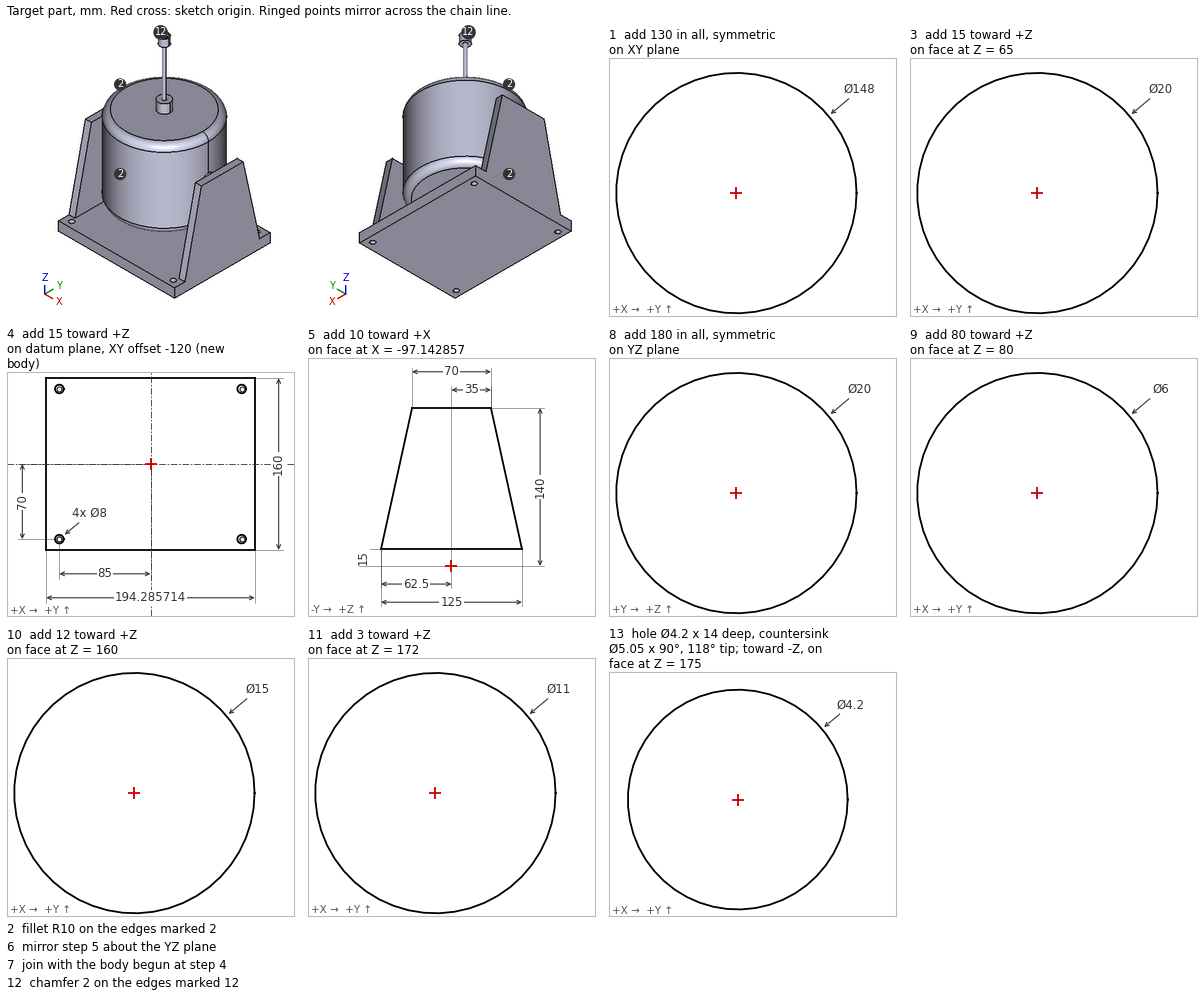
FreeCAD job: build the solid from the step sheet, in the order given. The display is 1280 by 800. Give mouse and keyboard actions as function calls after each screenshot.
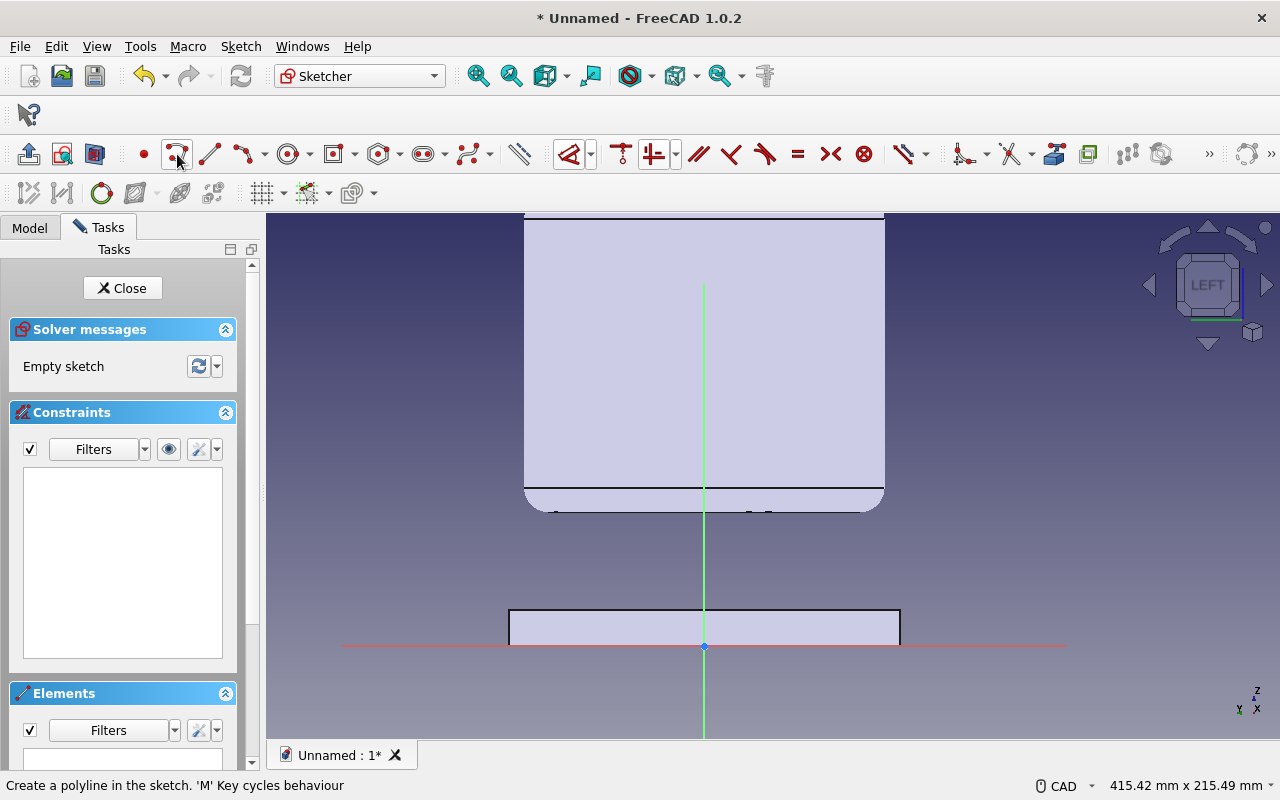
click(552, 610)
click(857, 610)
click(790, 305)
click(619, 305)
click(552, 611)
key(Escape)
key(Escape)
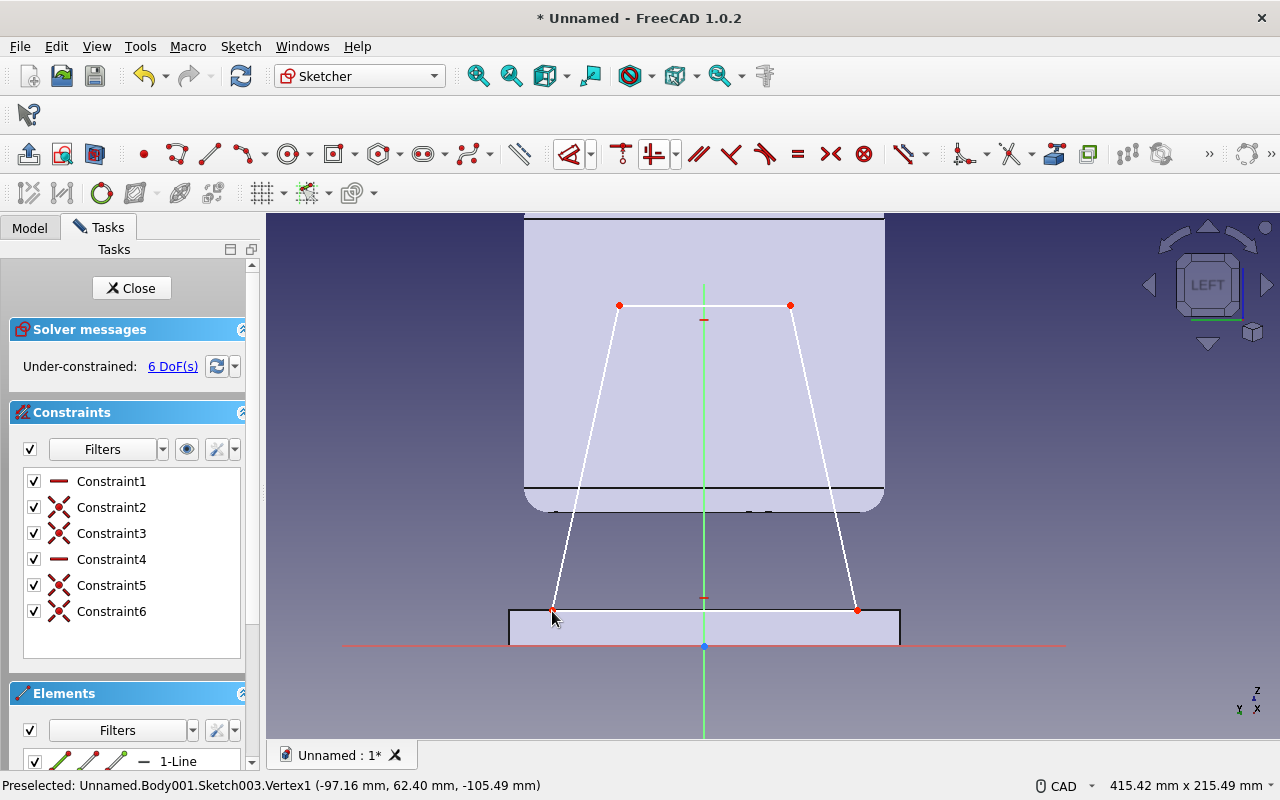
click(739, 306)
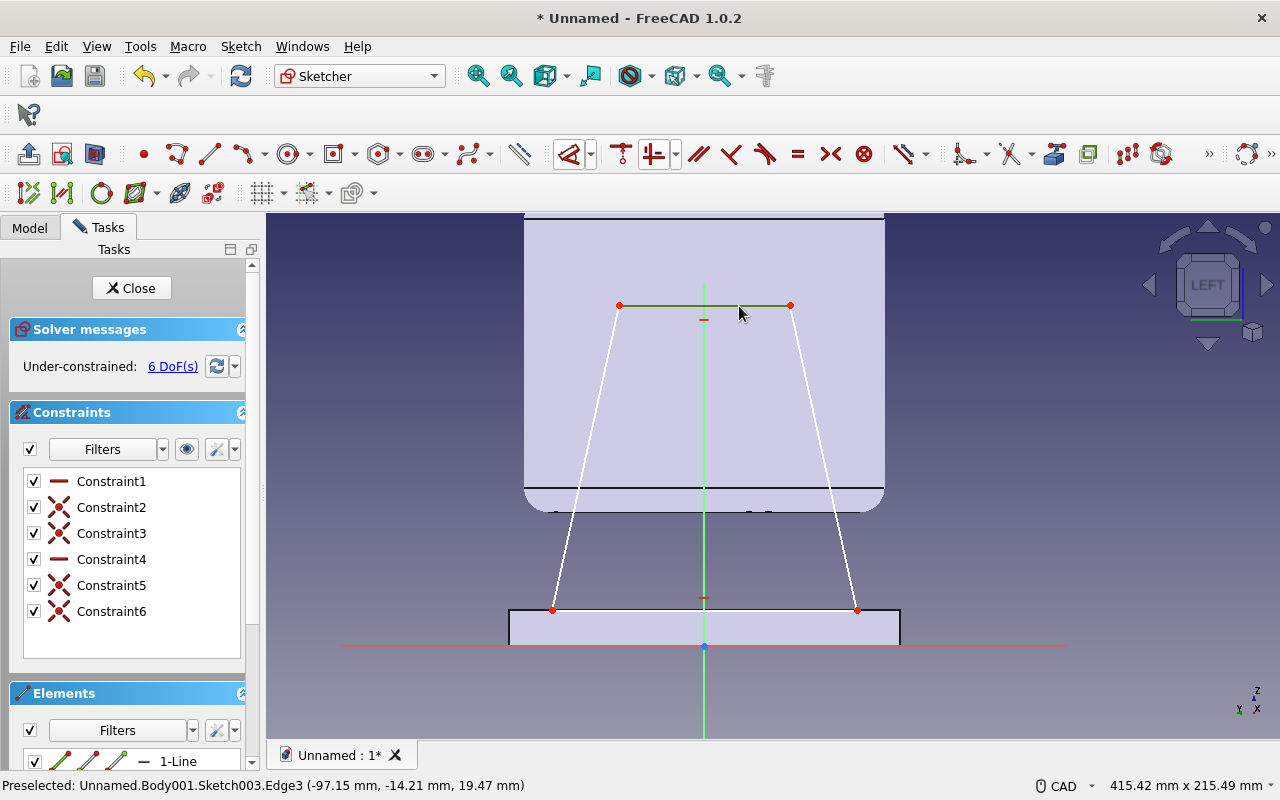
key(l)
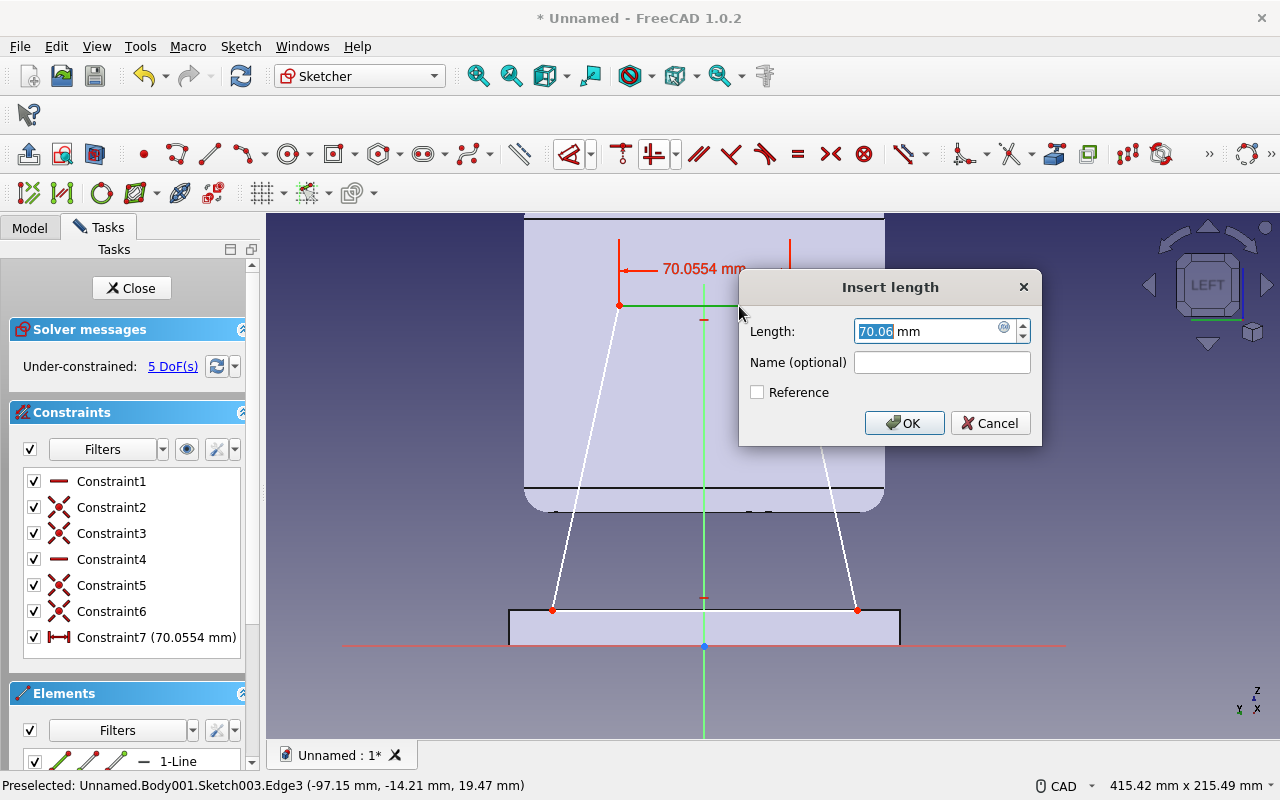
text(70)
key(Return)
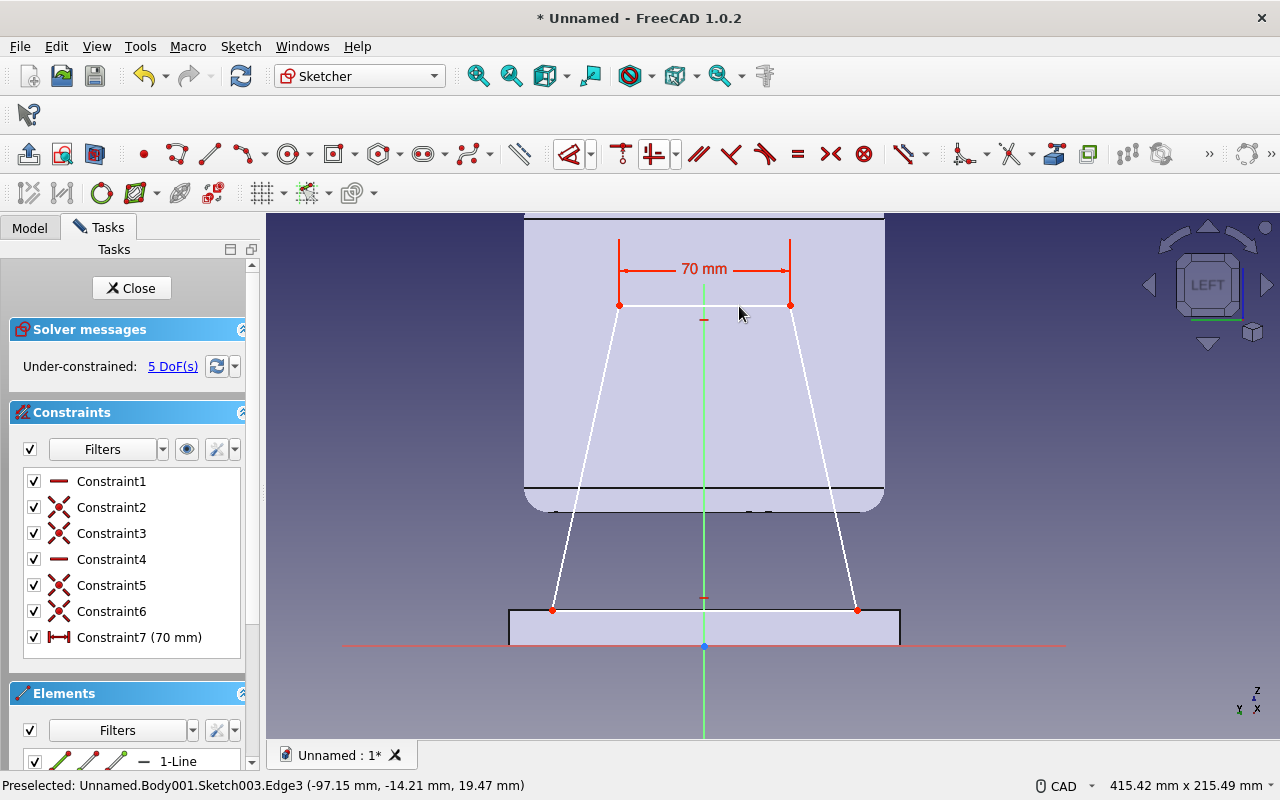
click(644, 611)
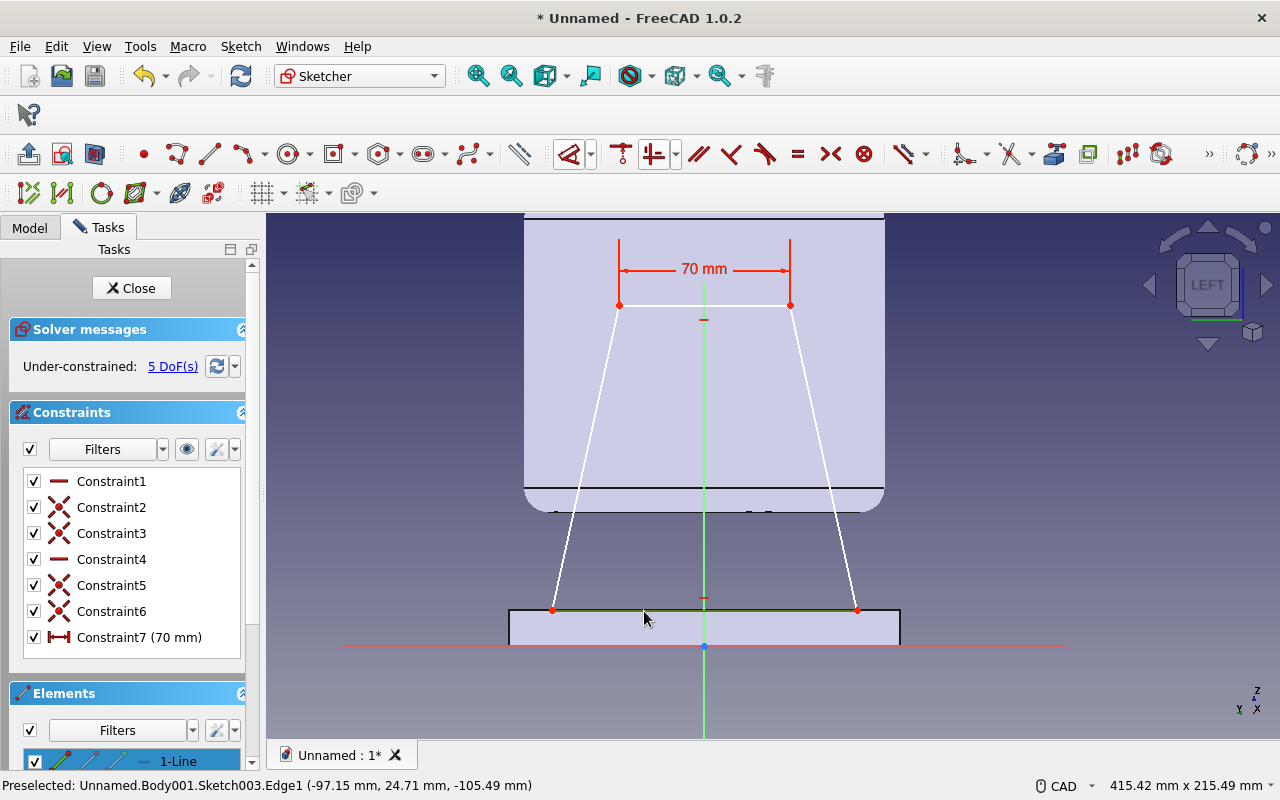
key(l)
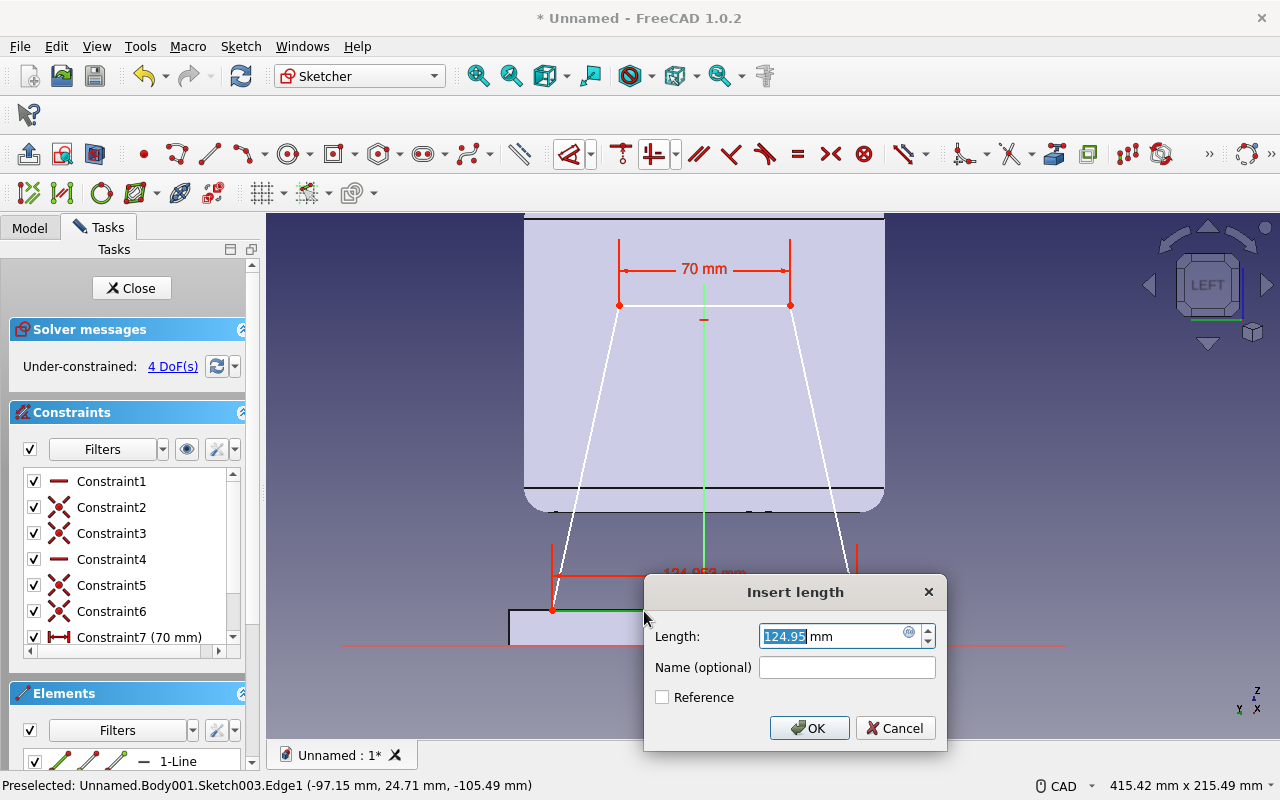
text(125)
key(Return)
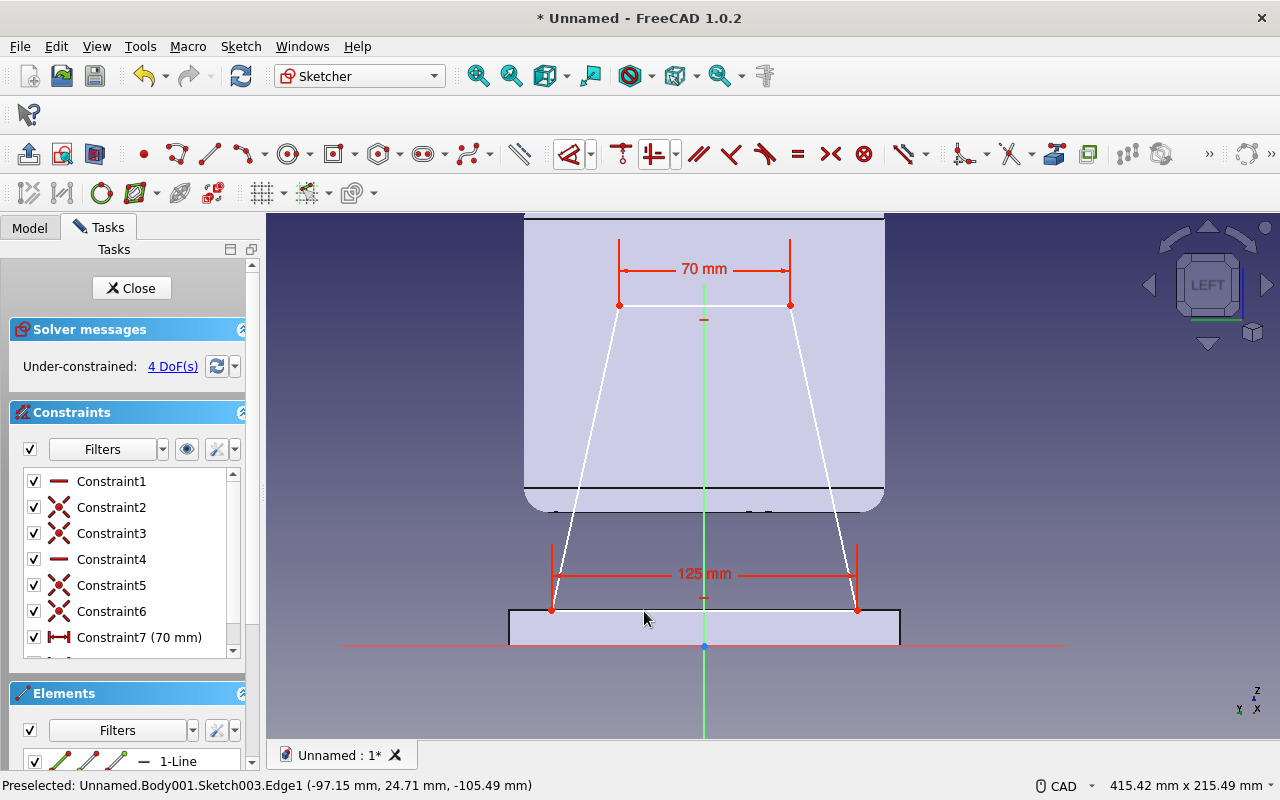
click(552, 611)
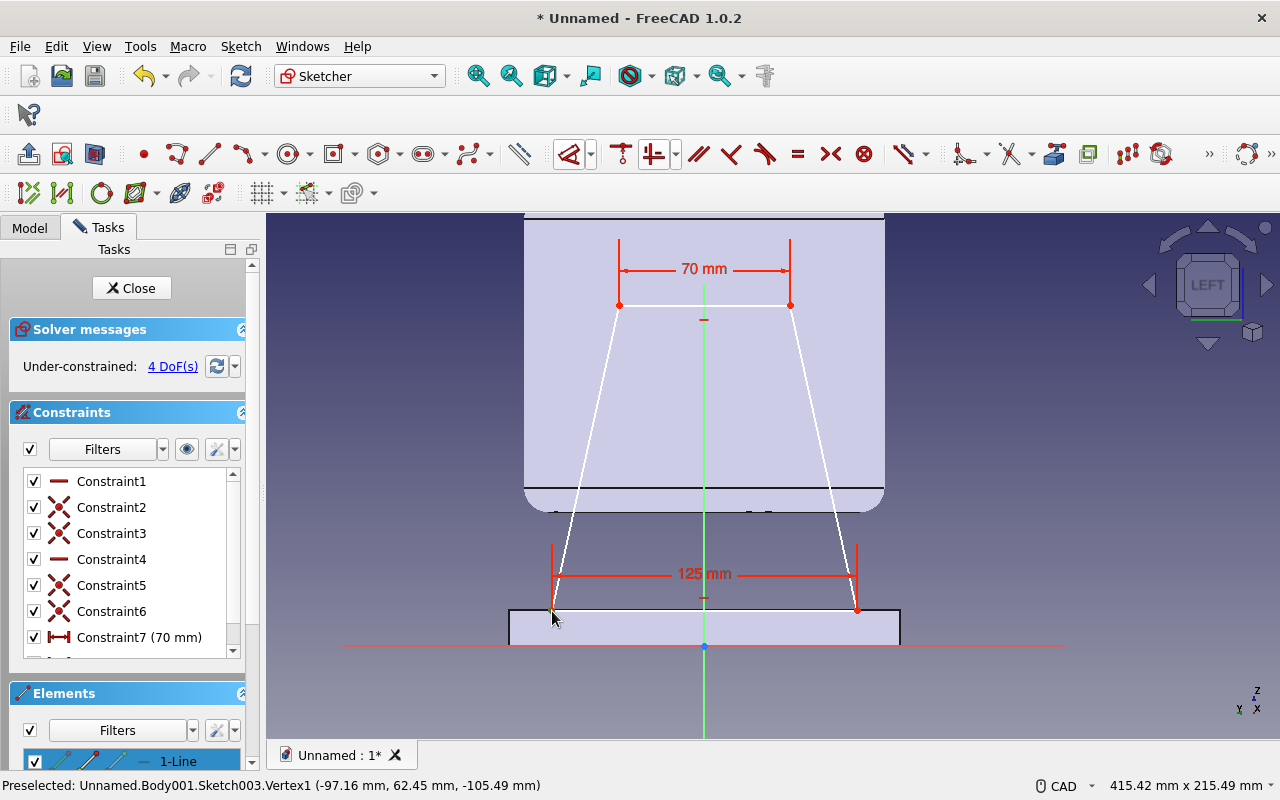
click(590, 154)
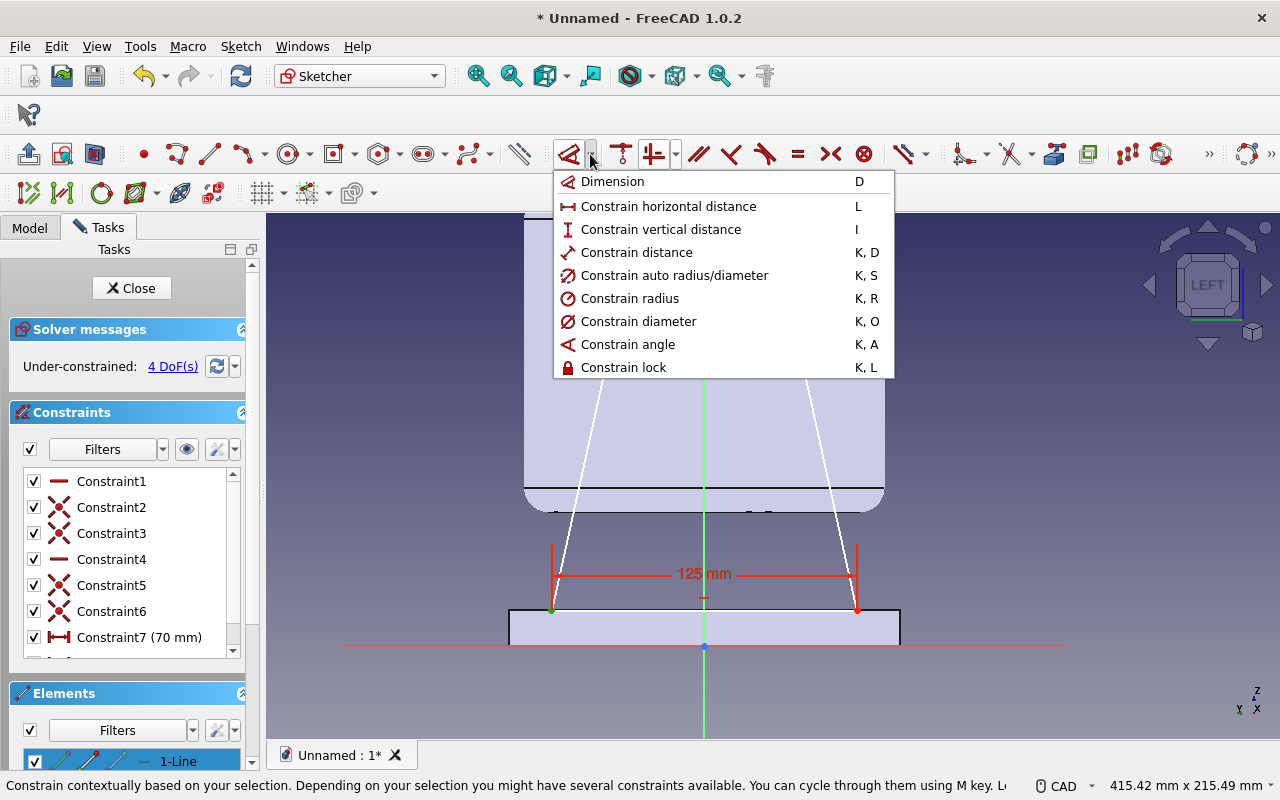
click(724, 230)